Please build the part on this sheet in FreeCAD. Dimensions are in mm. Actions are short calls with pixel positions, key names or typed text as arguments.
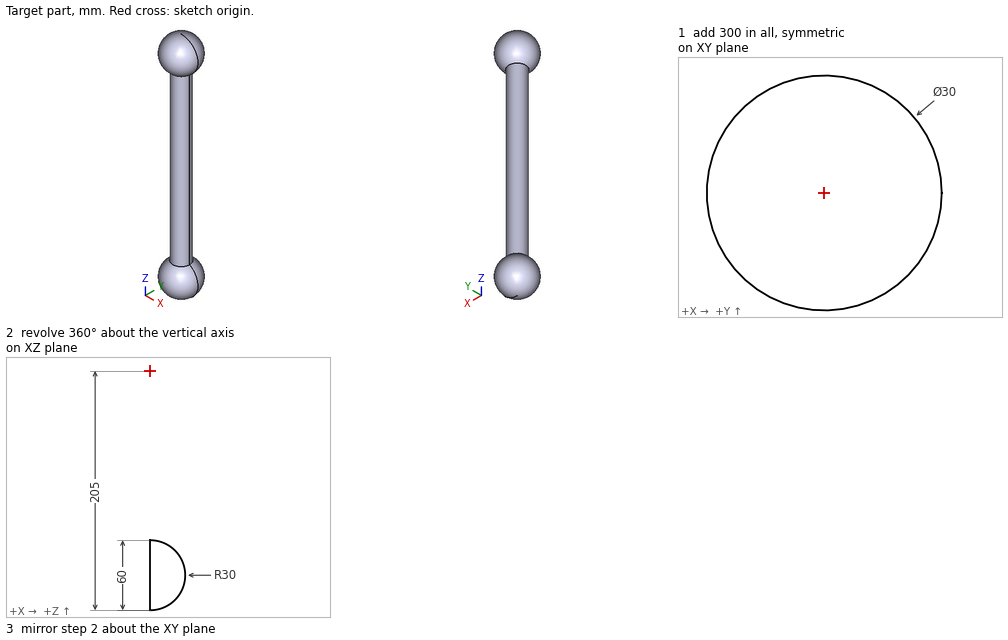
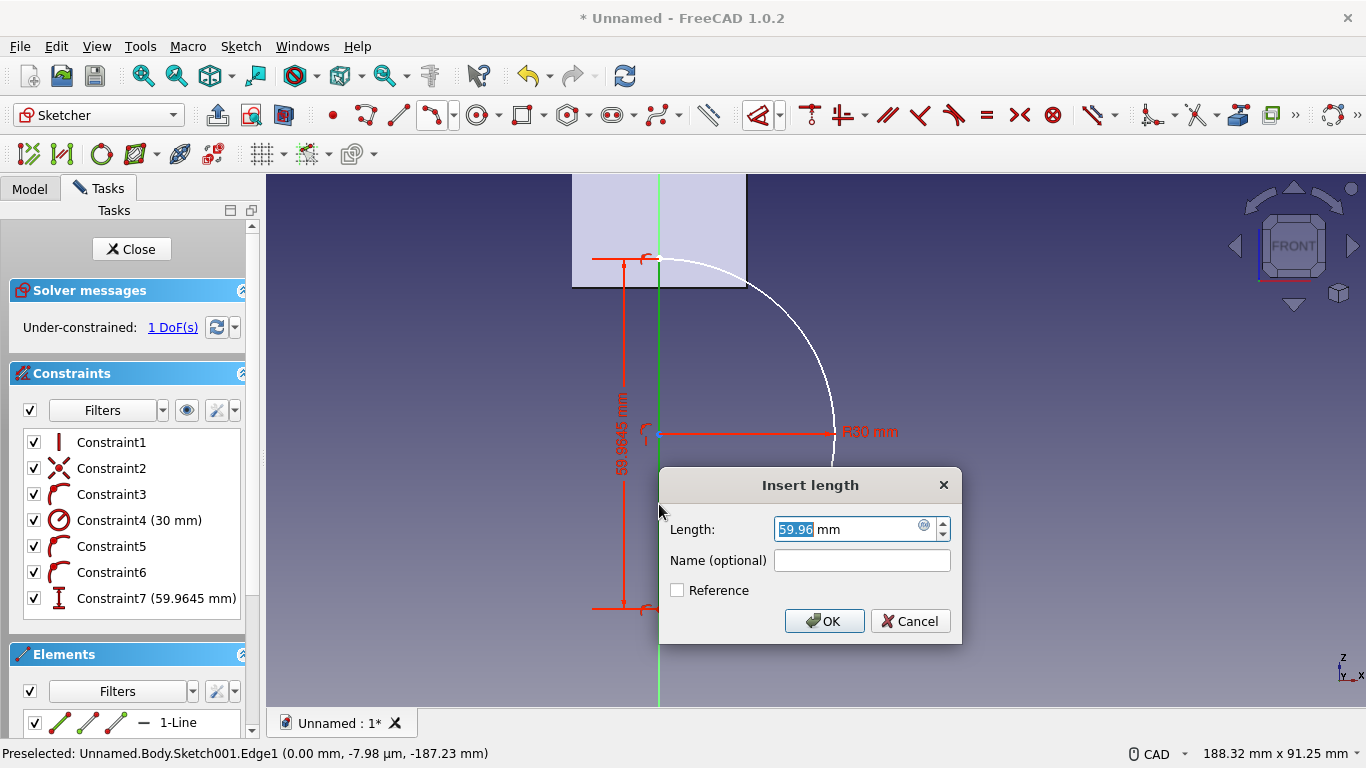
text(60)
key(Return)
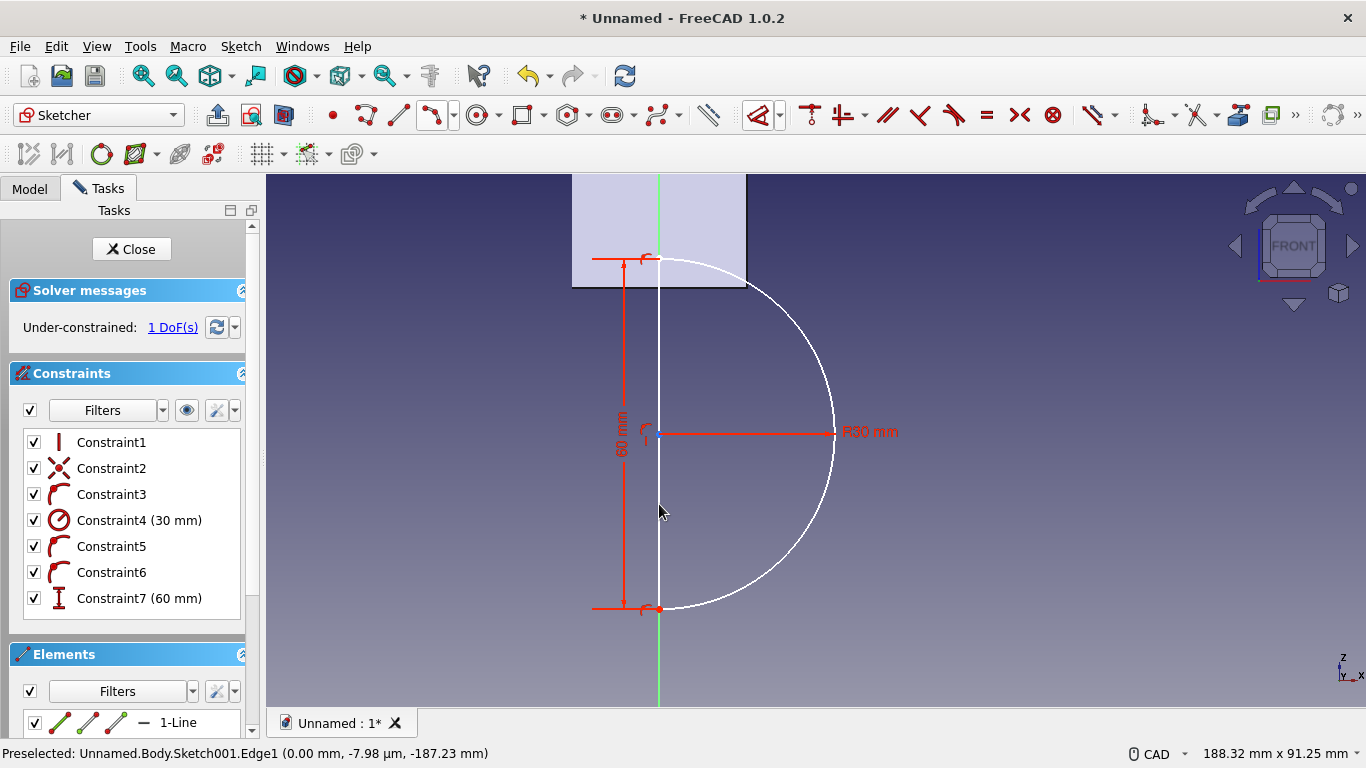
click(659, 609)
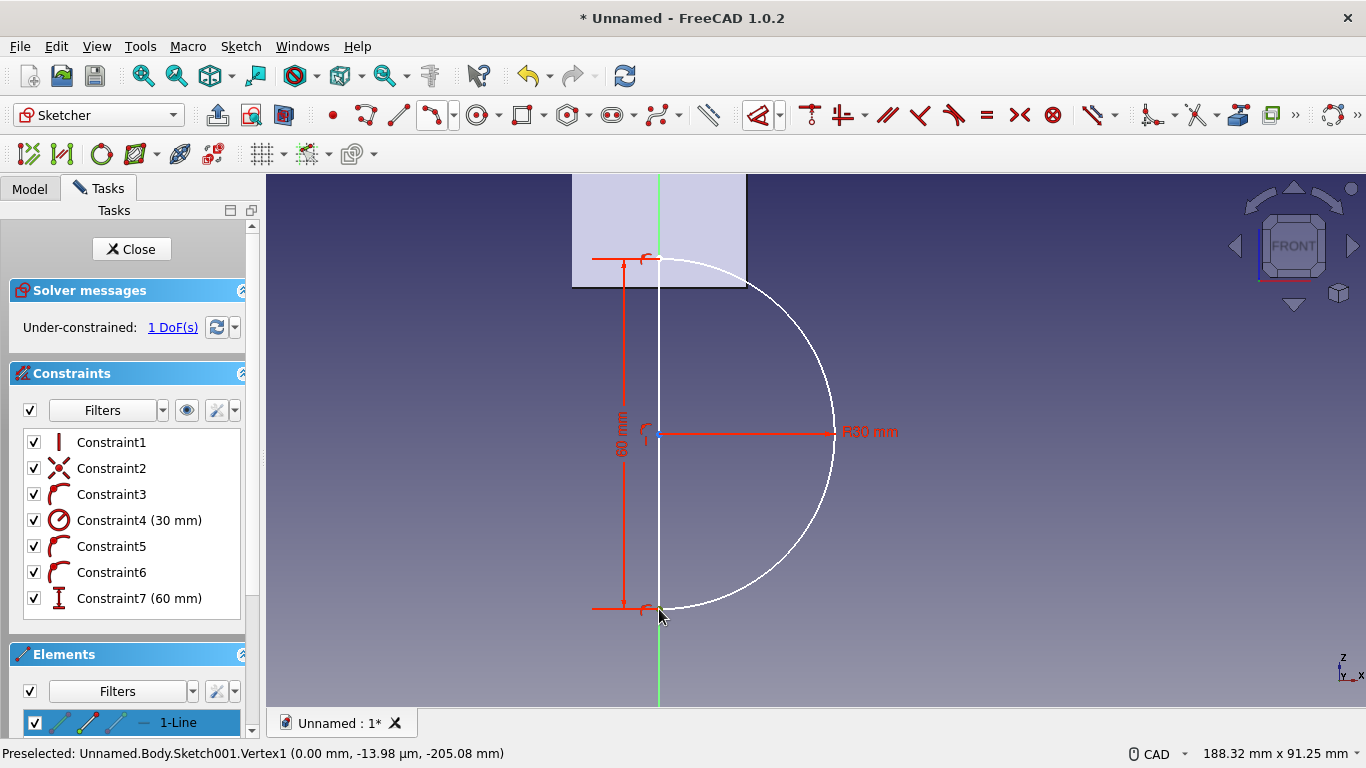
click(780, 116)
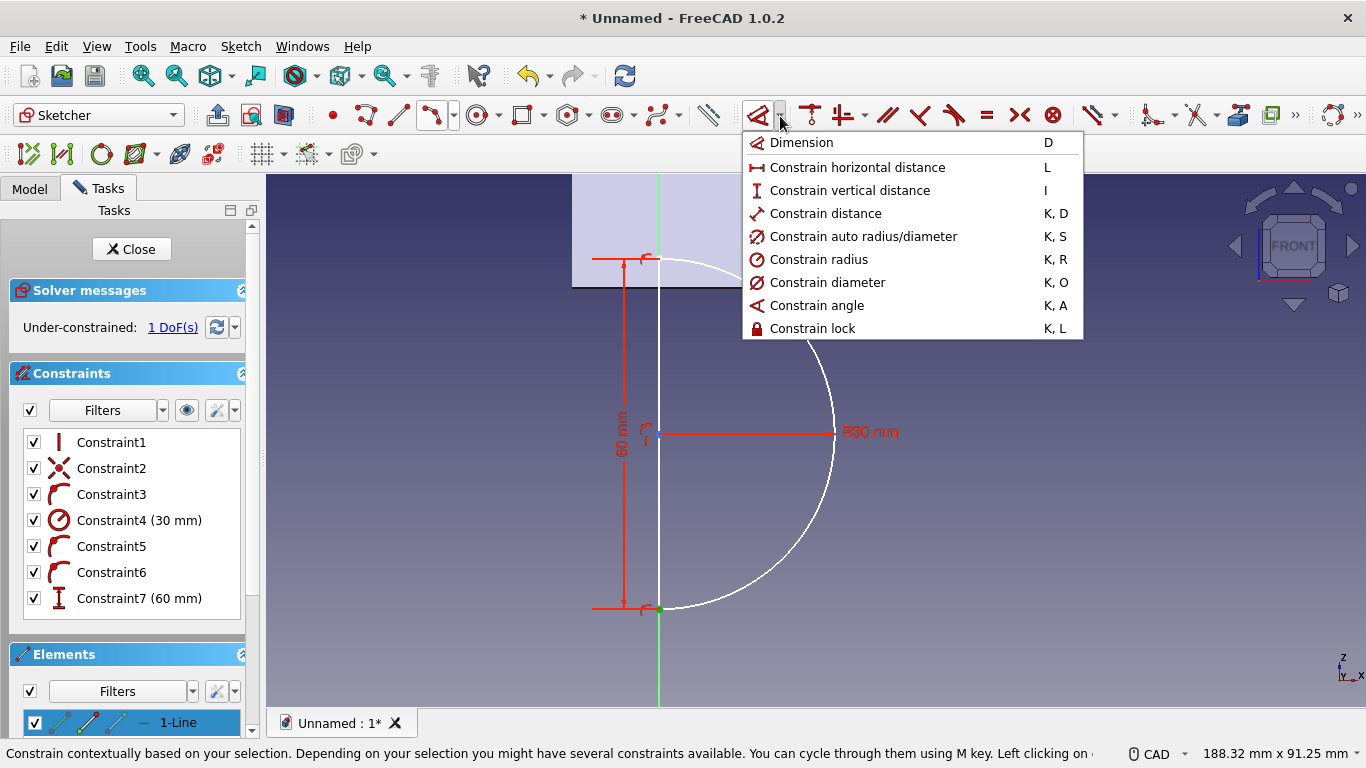
click(913, 190)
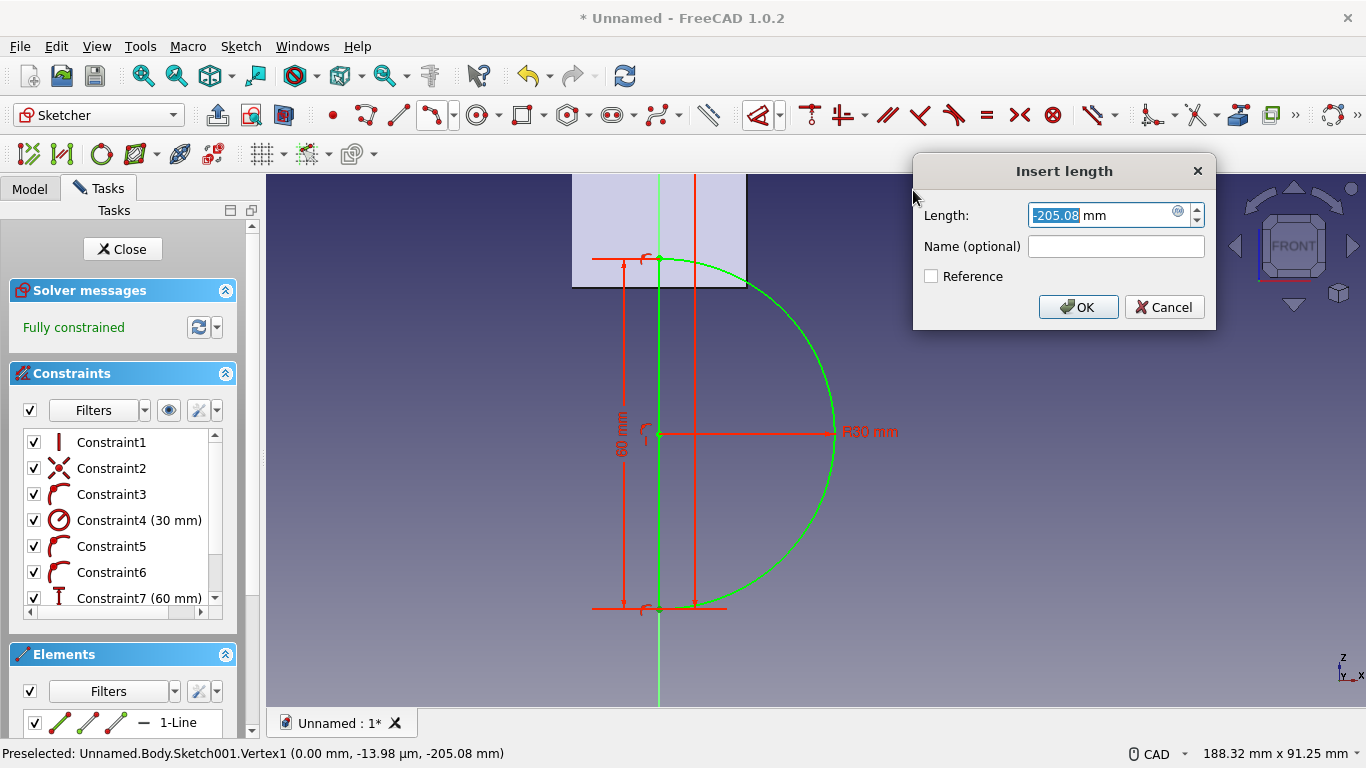
text(-205)
key(Return)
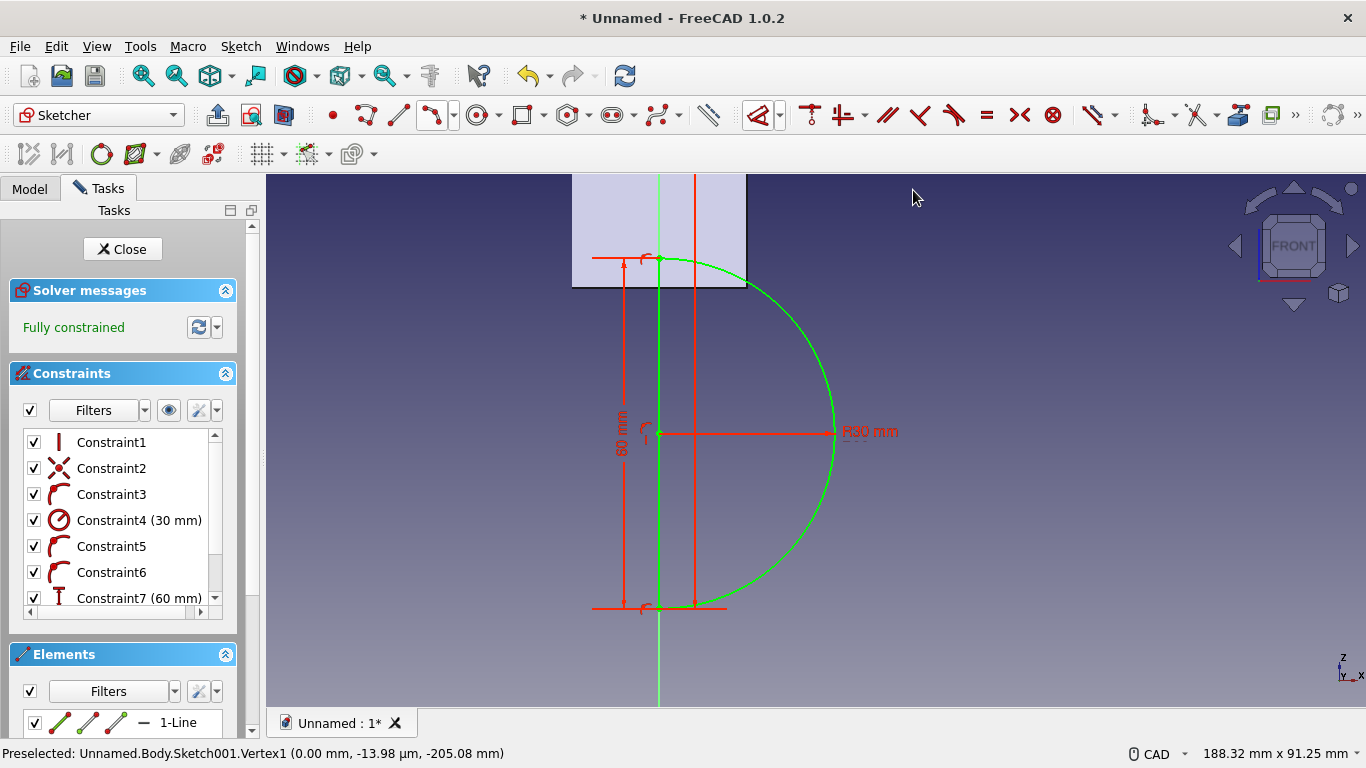
click(123, 249)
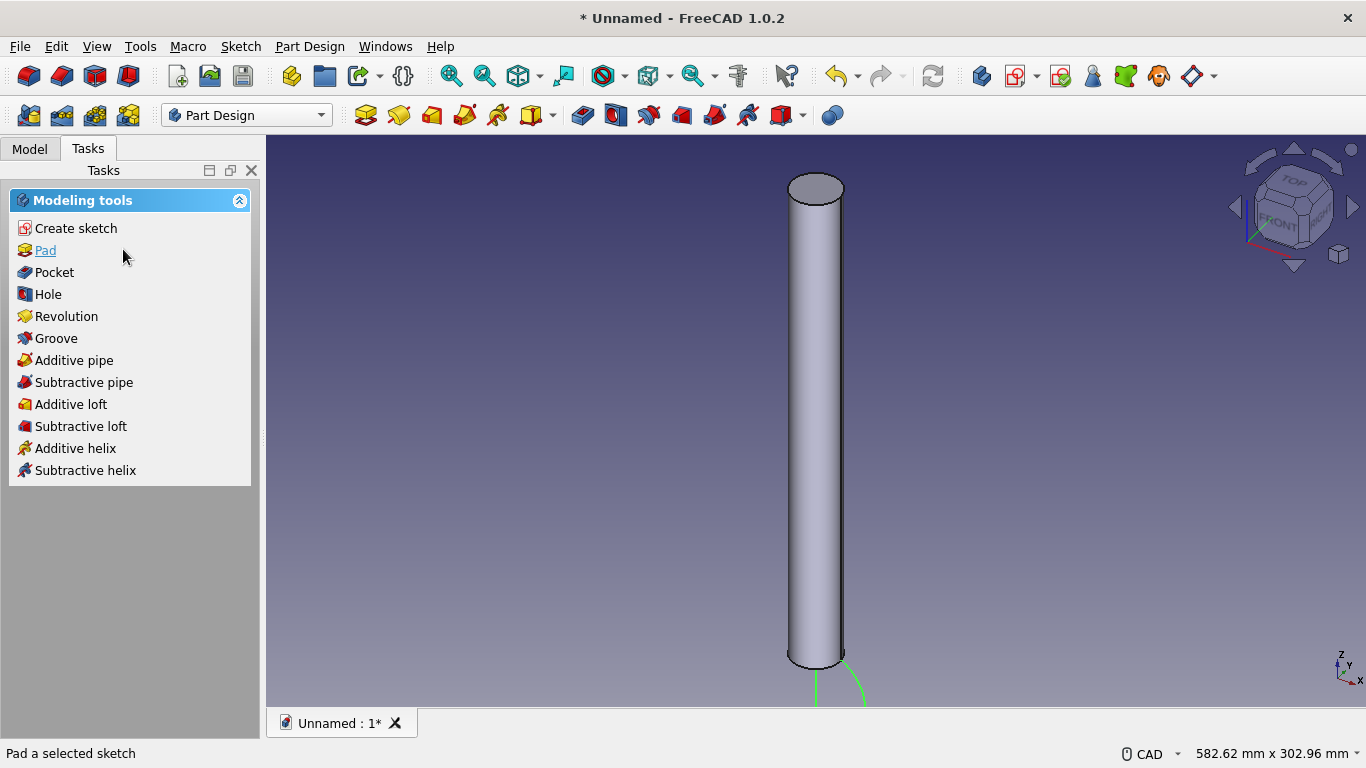
click(399, 116)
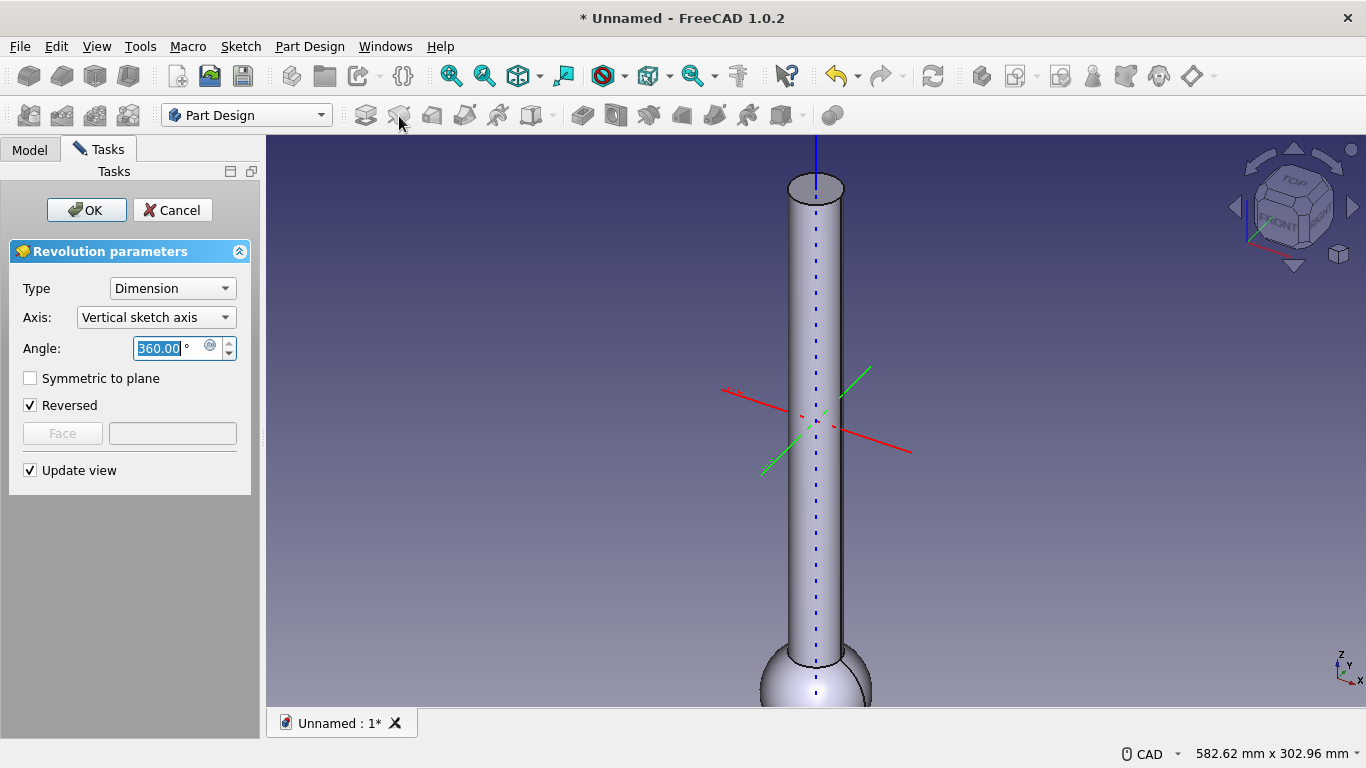
click(87, 210)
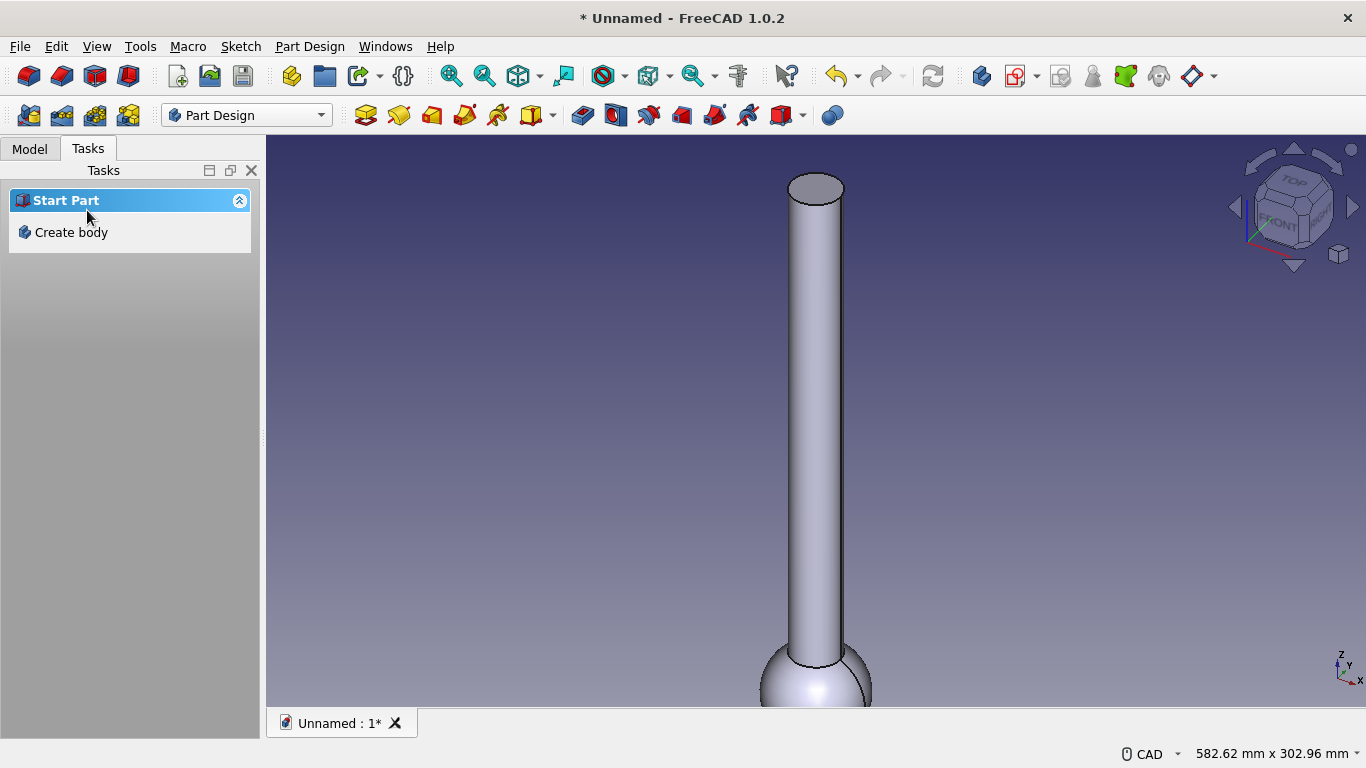
click(452, 76)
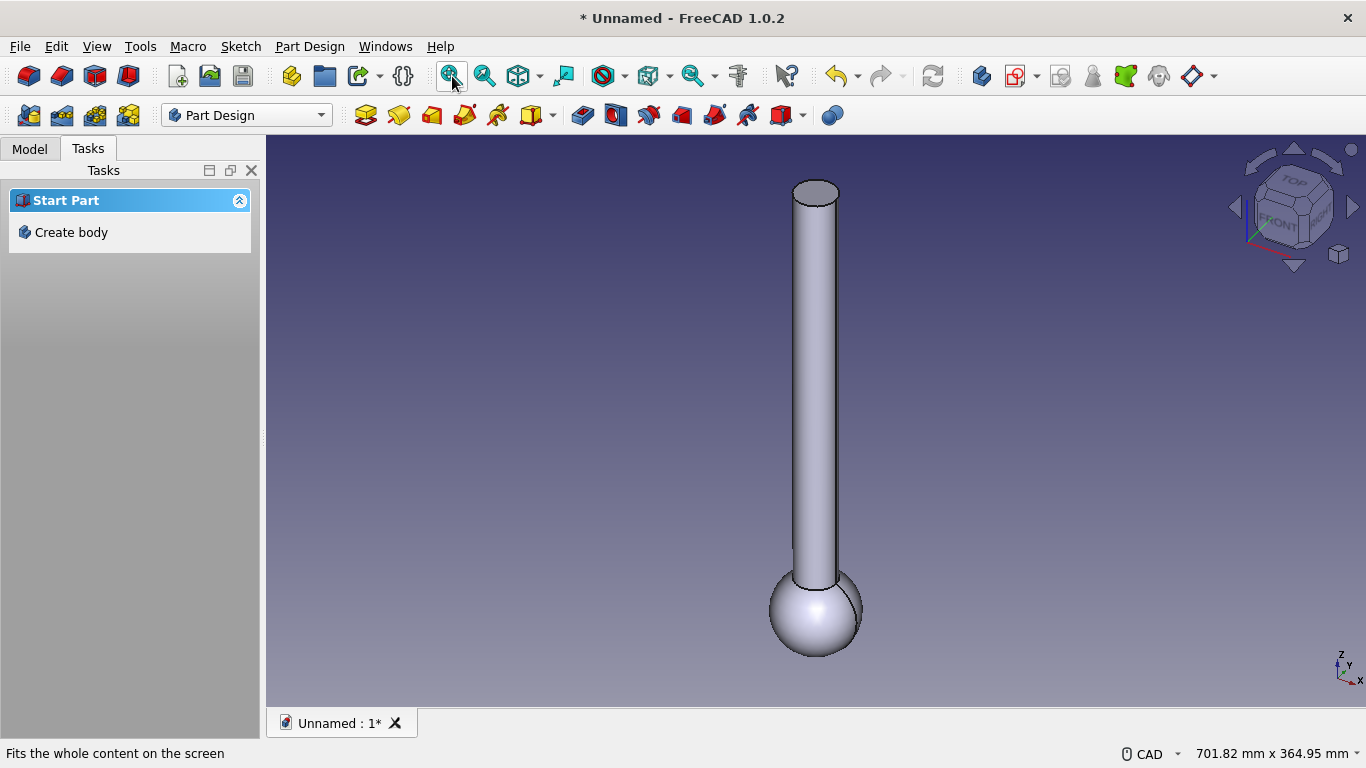
click(30, 148)